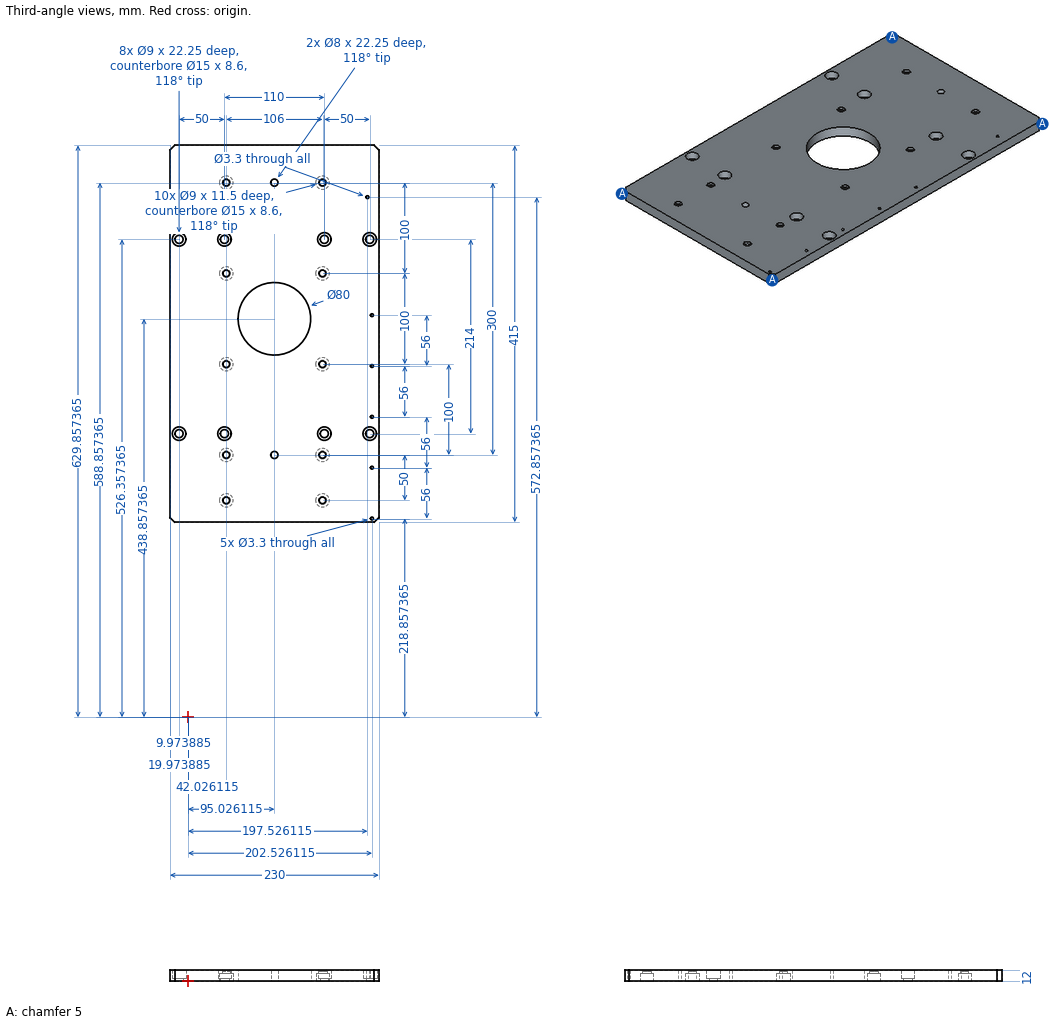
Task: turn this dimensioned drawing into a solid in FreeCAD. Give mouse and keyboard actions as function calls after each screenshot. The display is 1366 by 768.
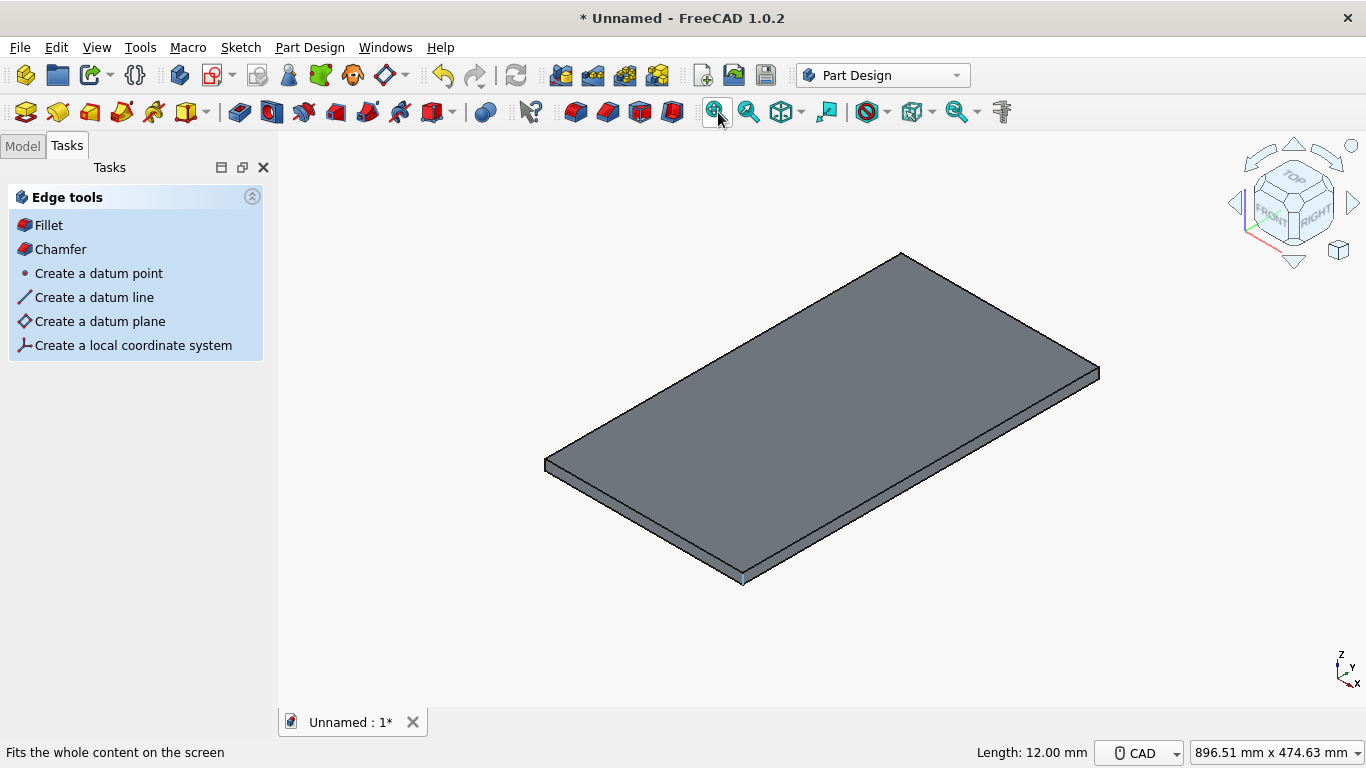
key(2)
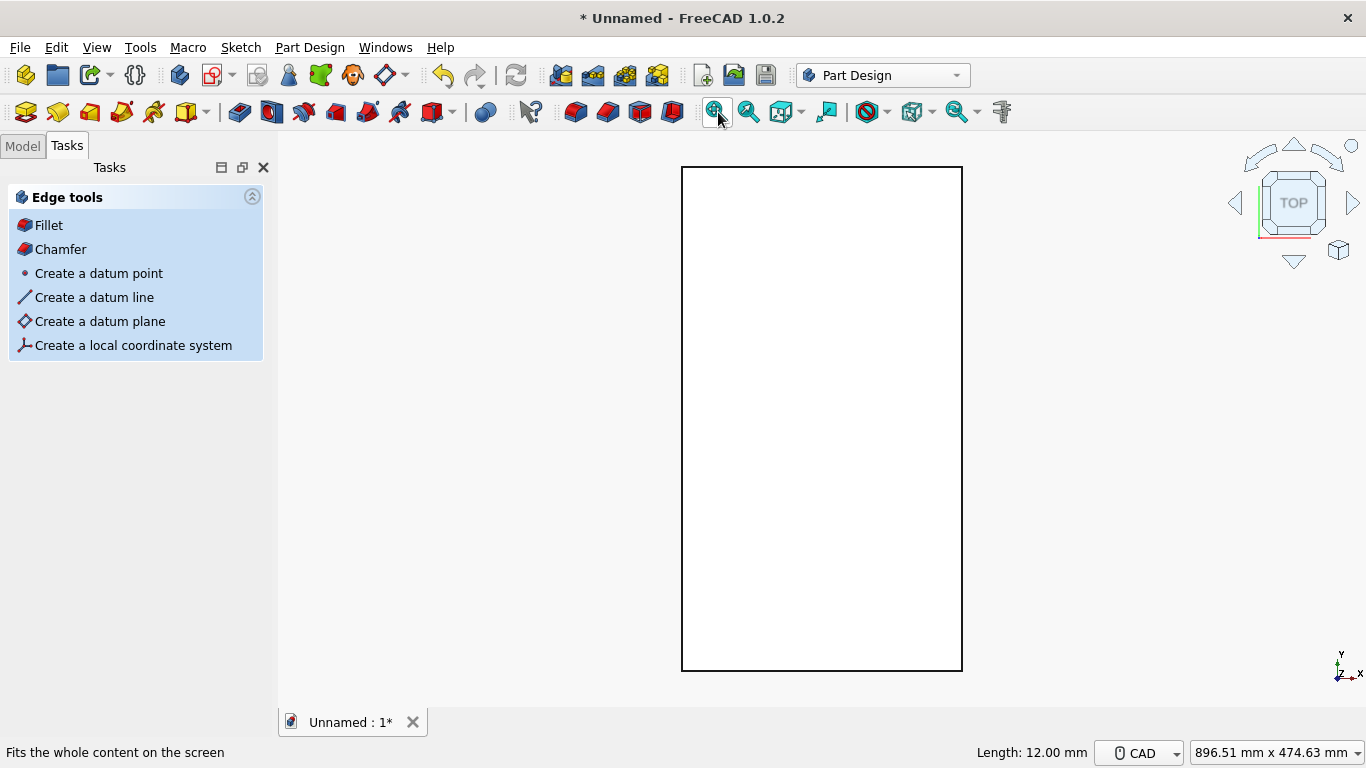
scroll(682, 670, up, 6)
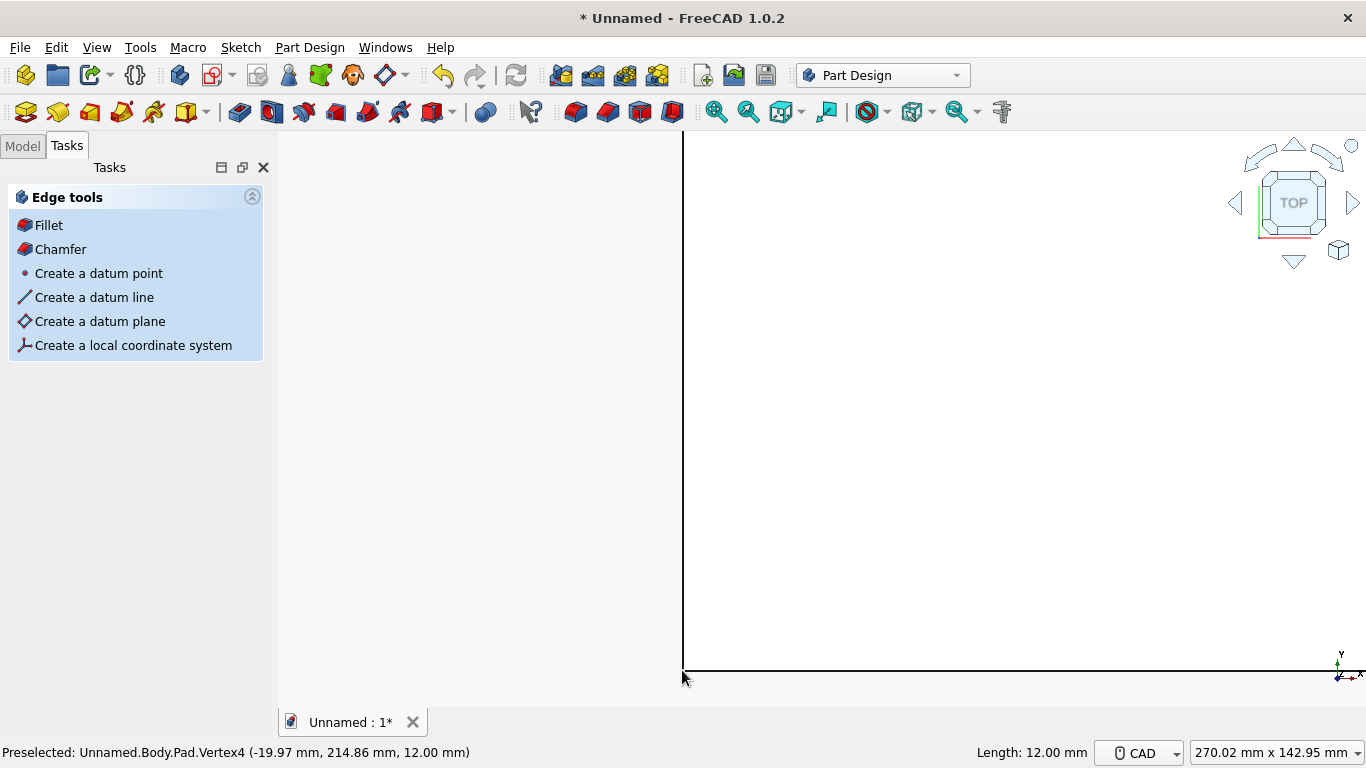
click(718, 112)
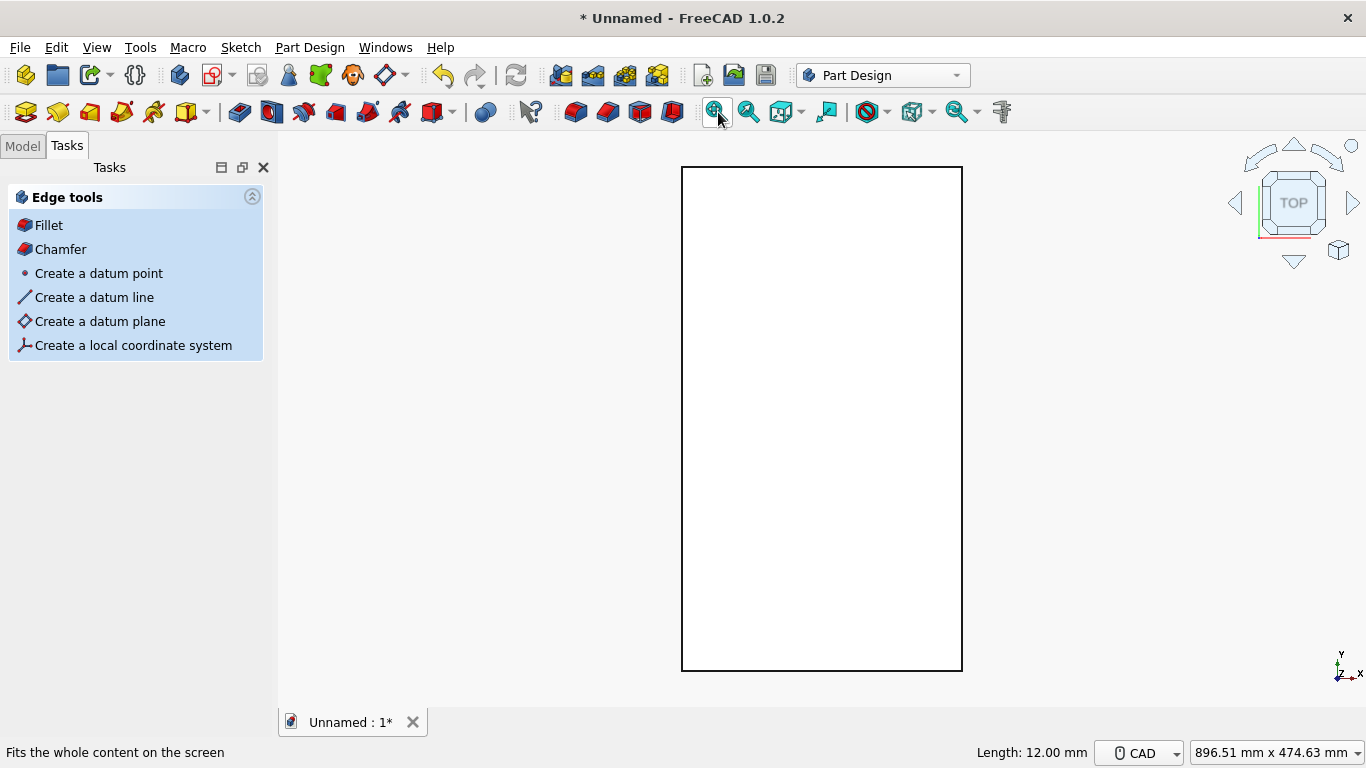
key(1)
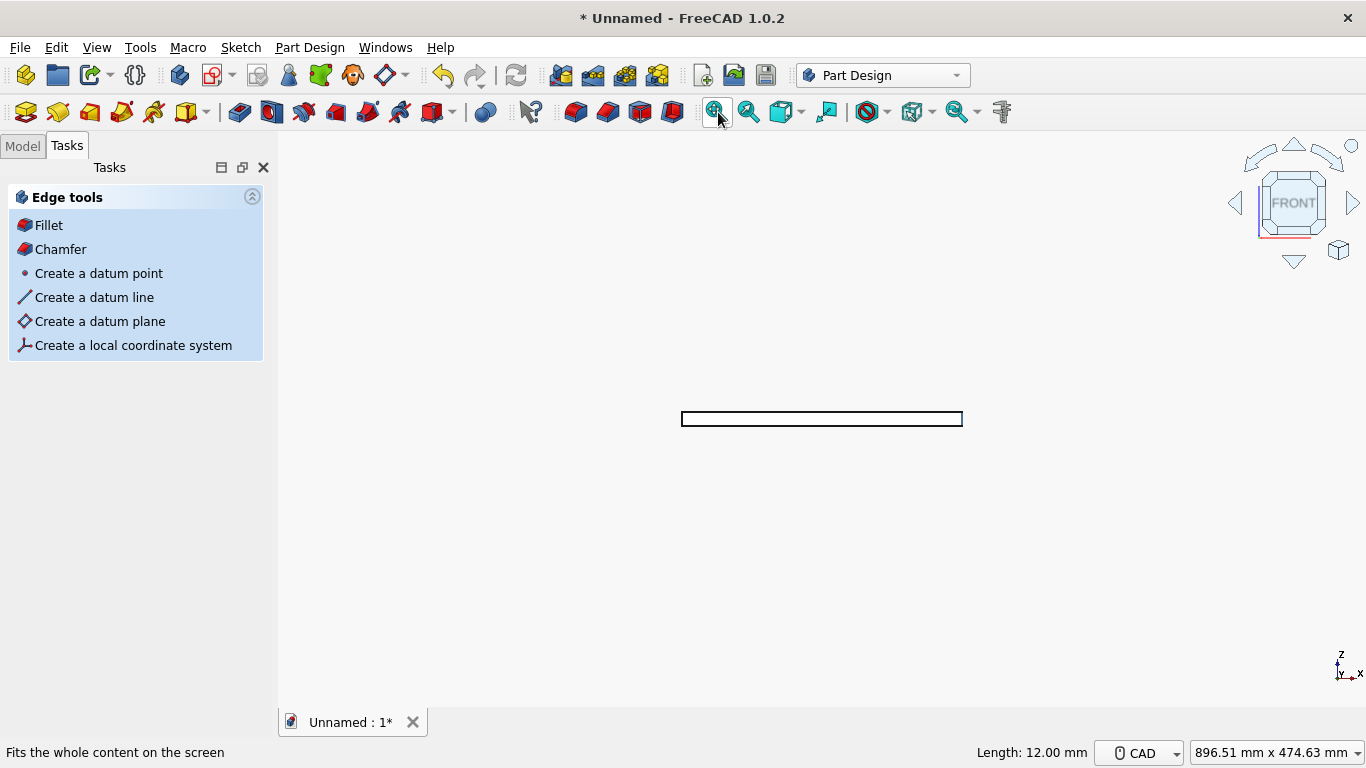
click(718, 112)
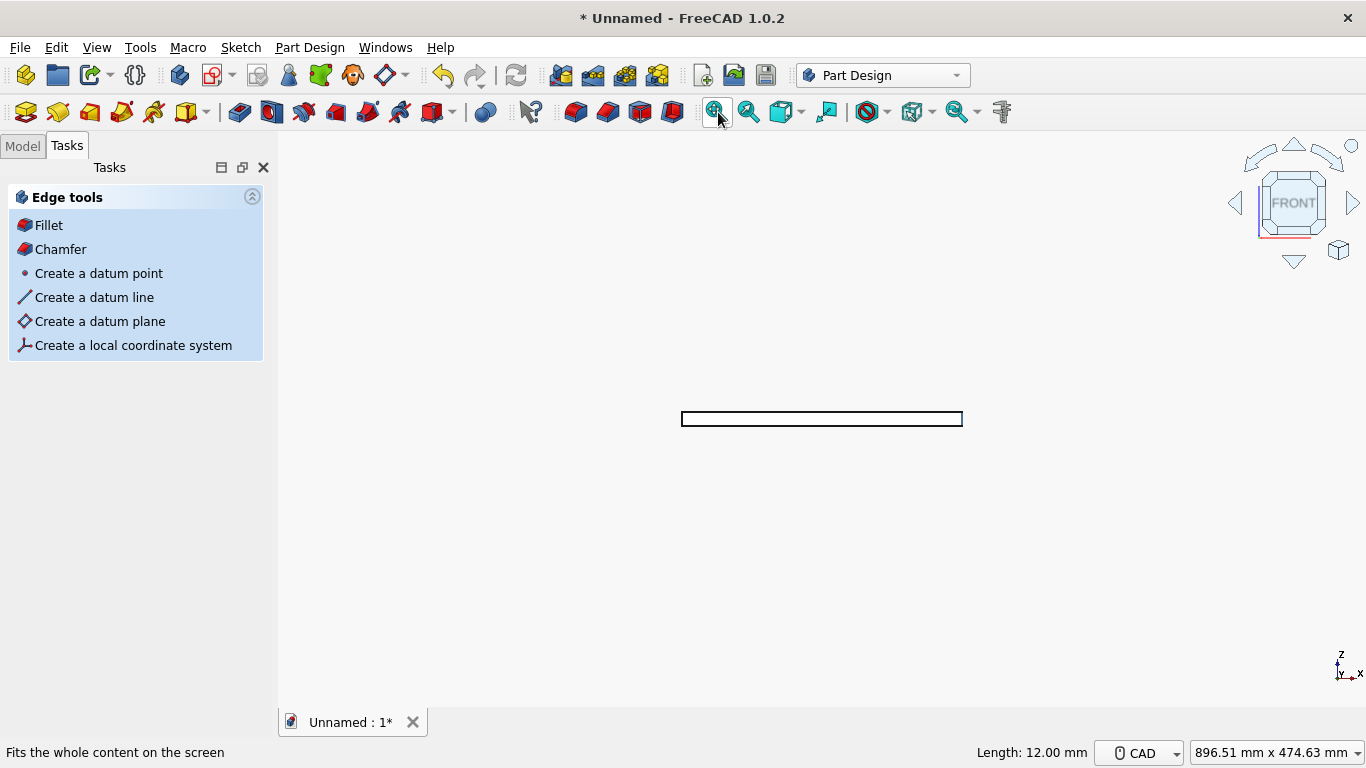
click(682, 418, ctrl)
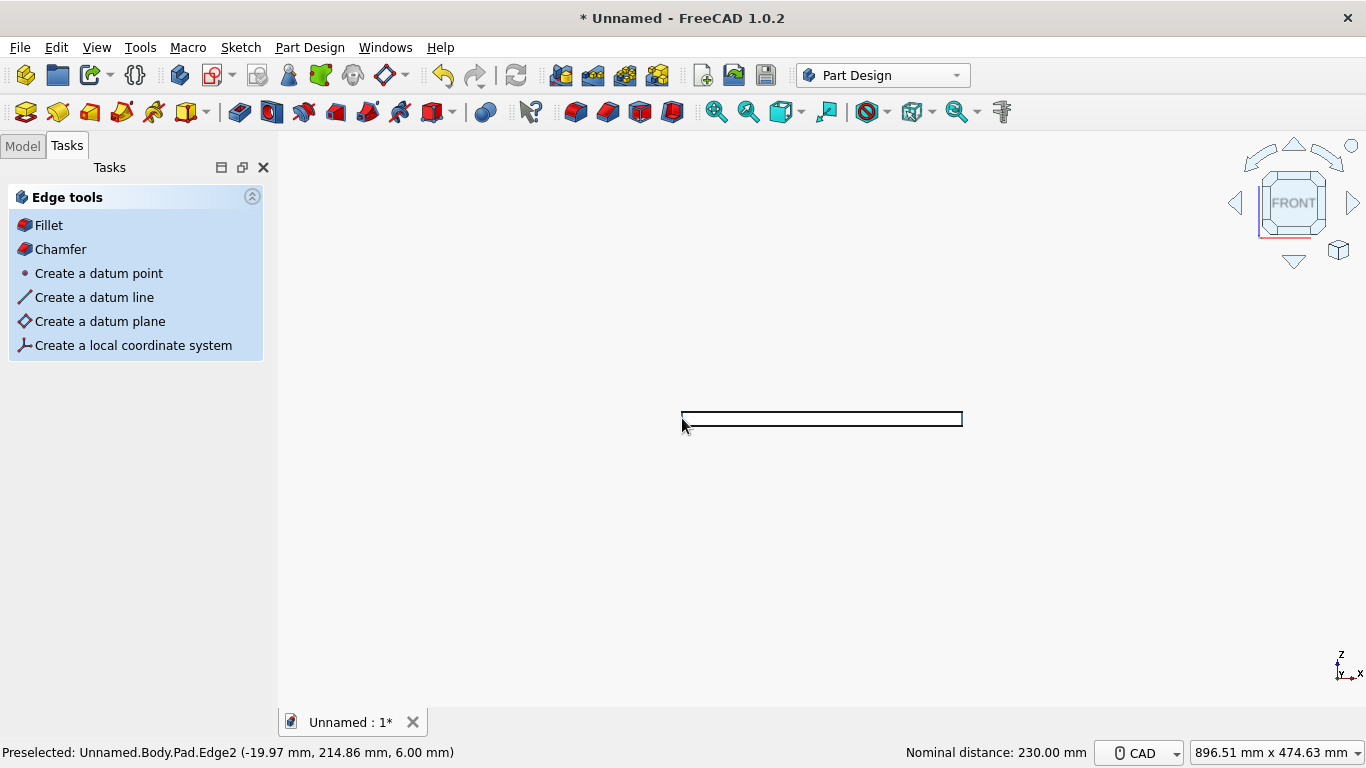
scroll(682, 418, up, 6)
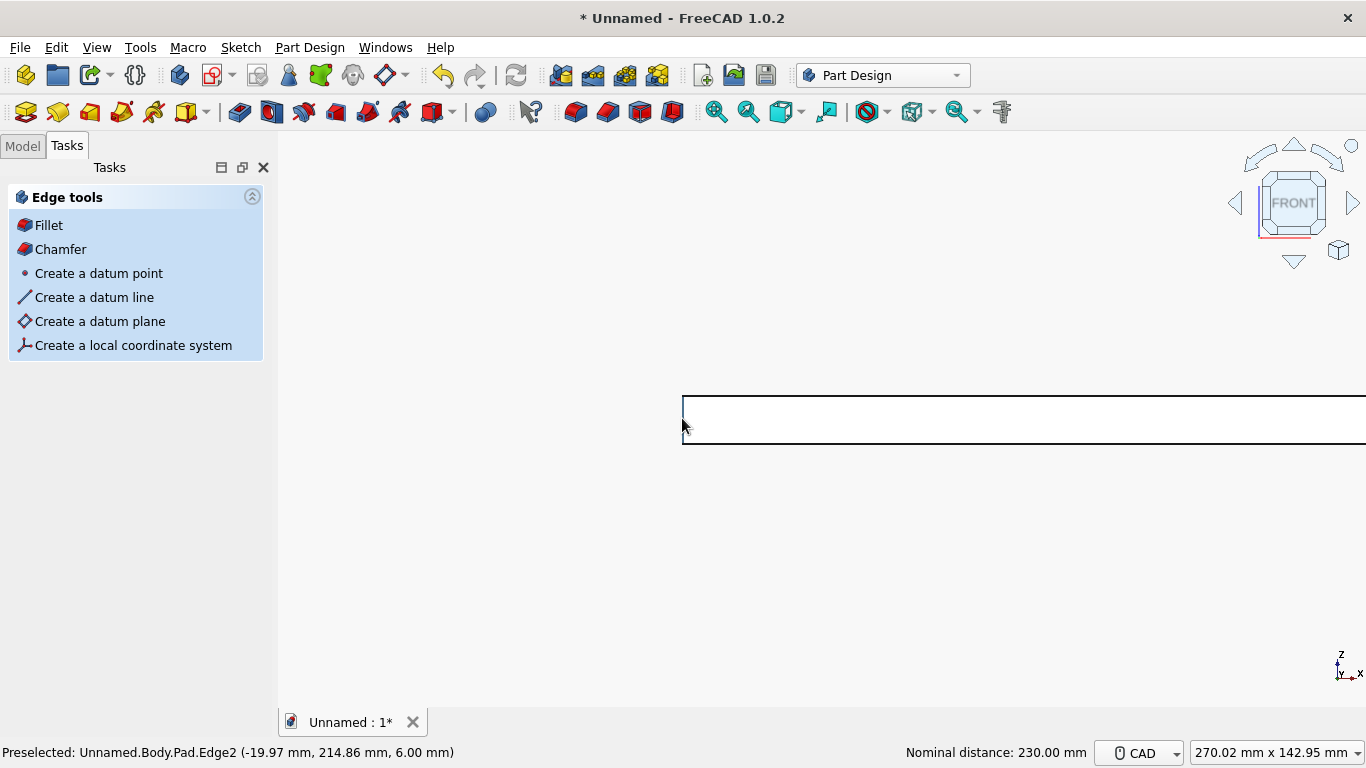
click(718, 112)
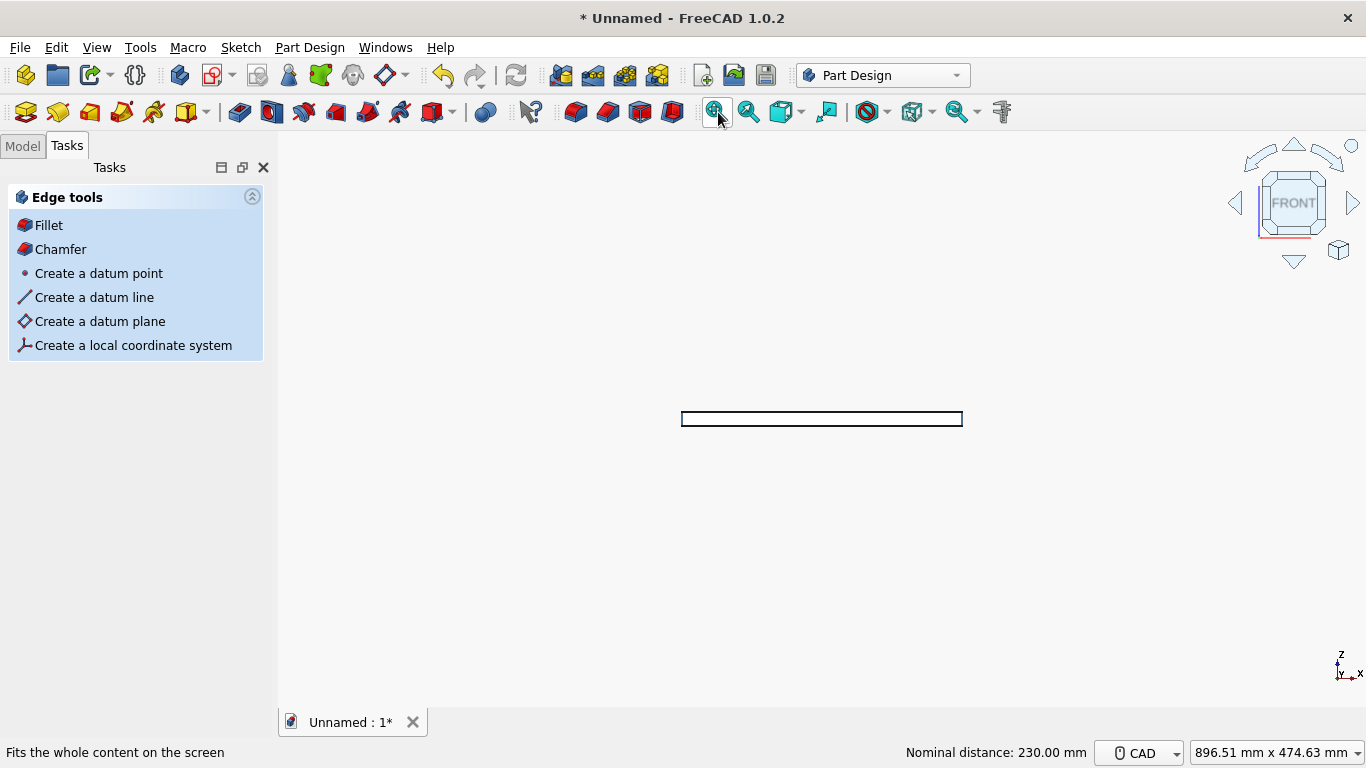
key(3)